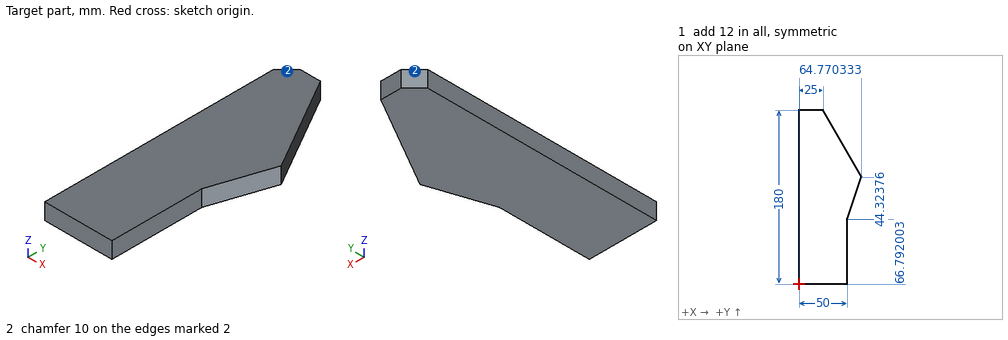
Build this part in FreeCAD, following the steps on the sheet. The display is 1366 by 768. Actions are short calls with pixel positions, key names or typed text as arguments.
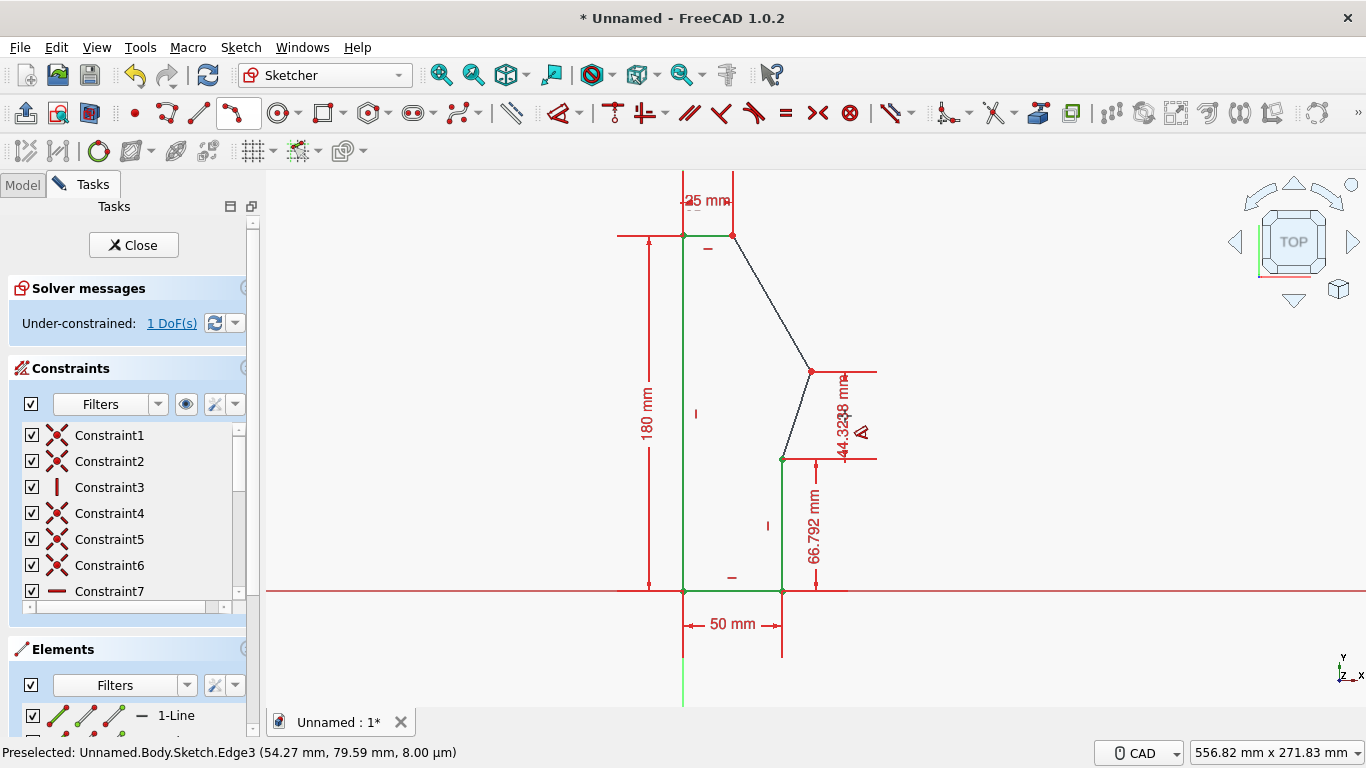
click(811, 372)
click(747, 338)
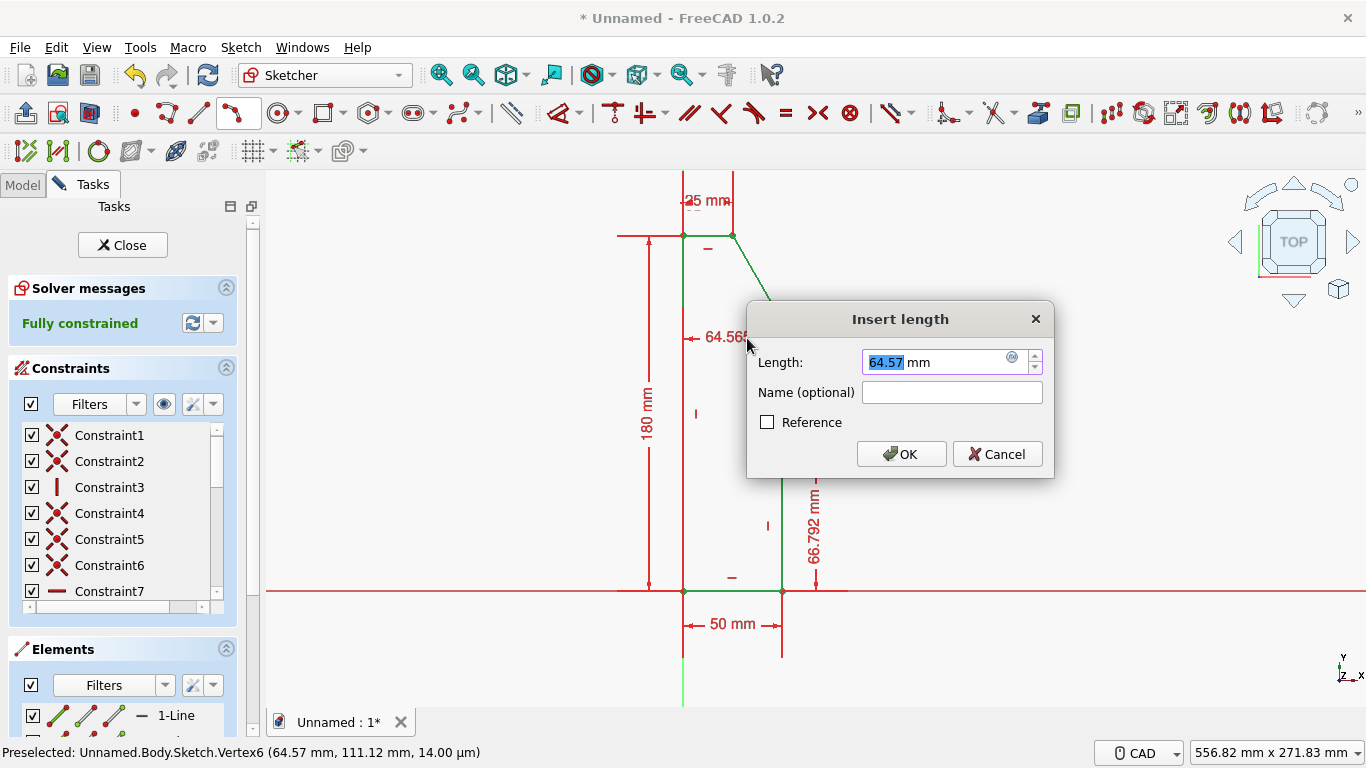
text(64.770333)
key(Return)
key(Escape)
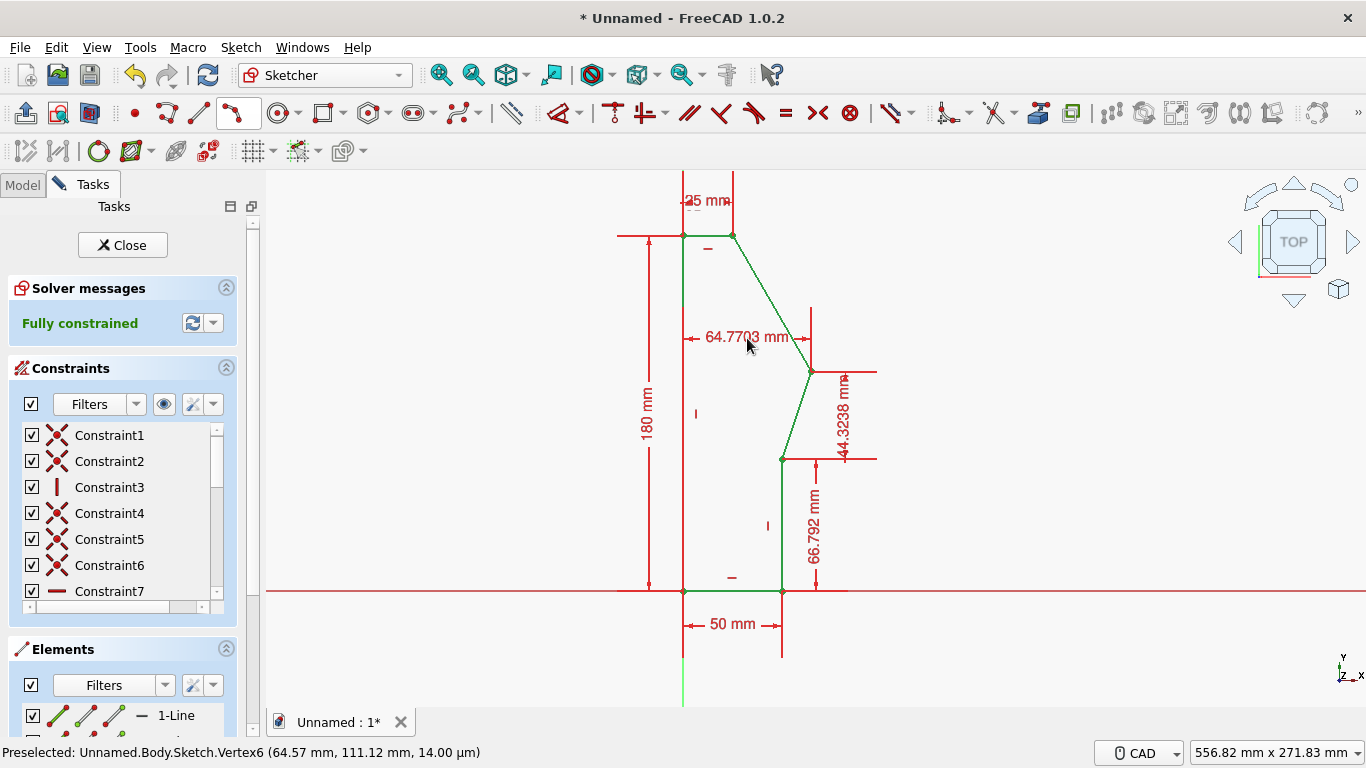
click(123, 245)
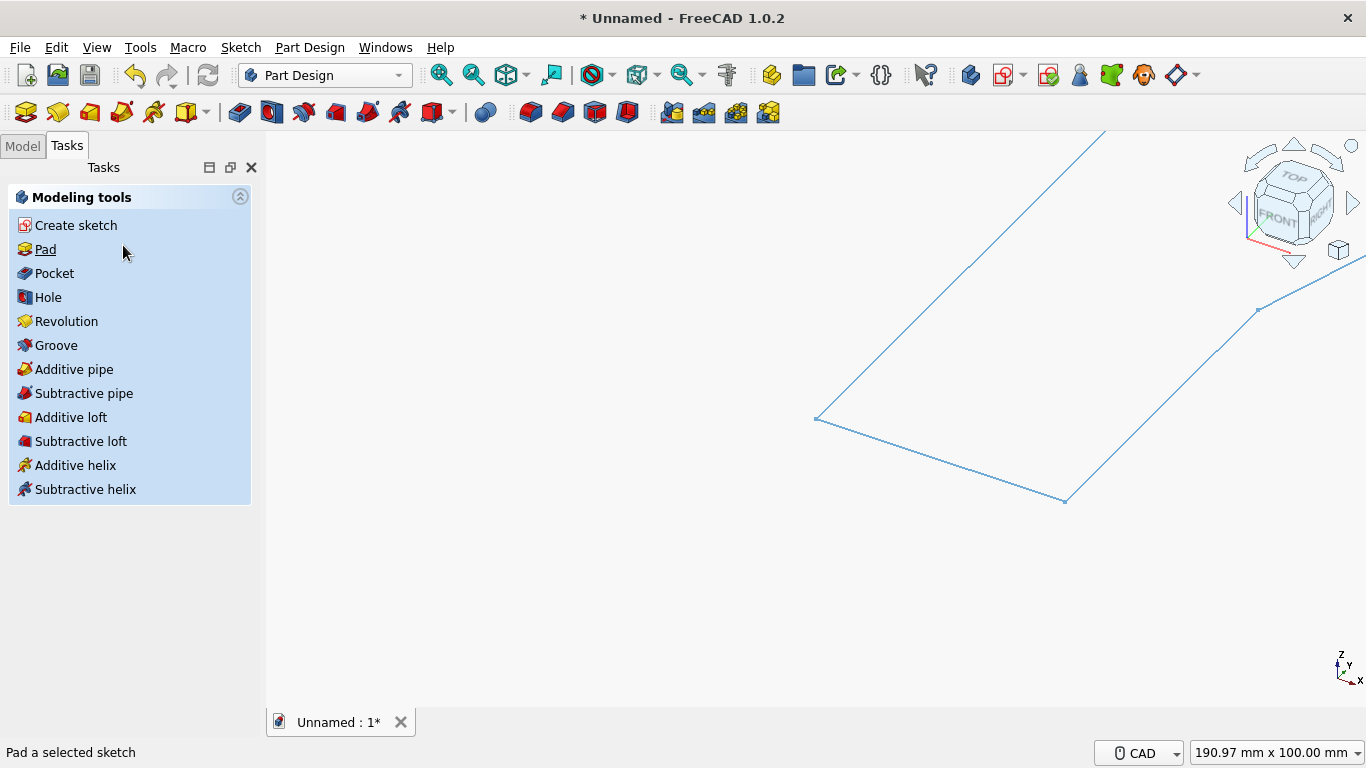
click(26, 112)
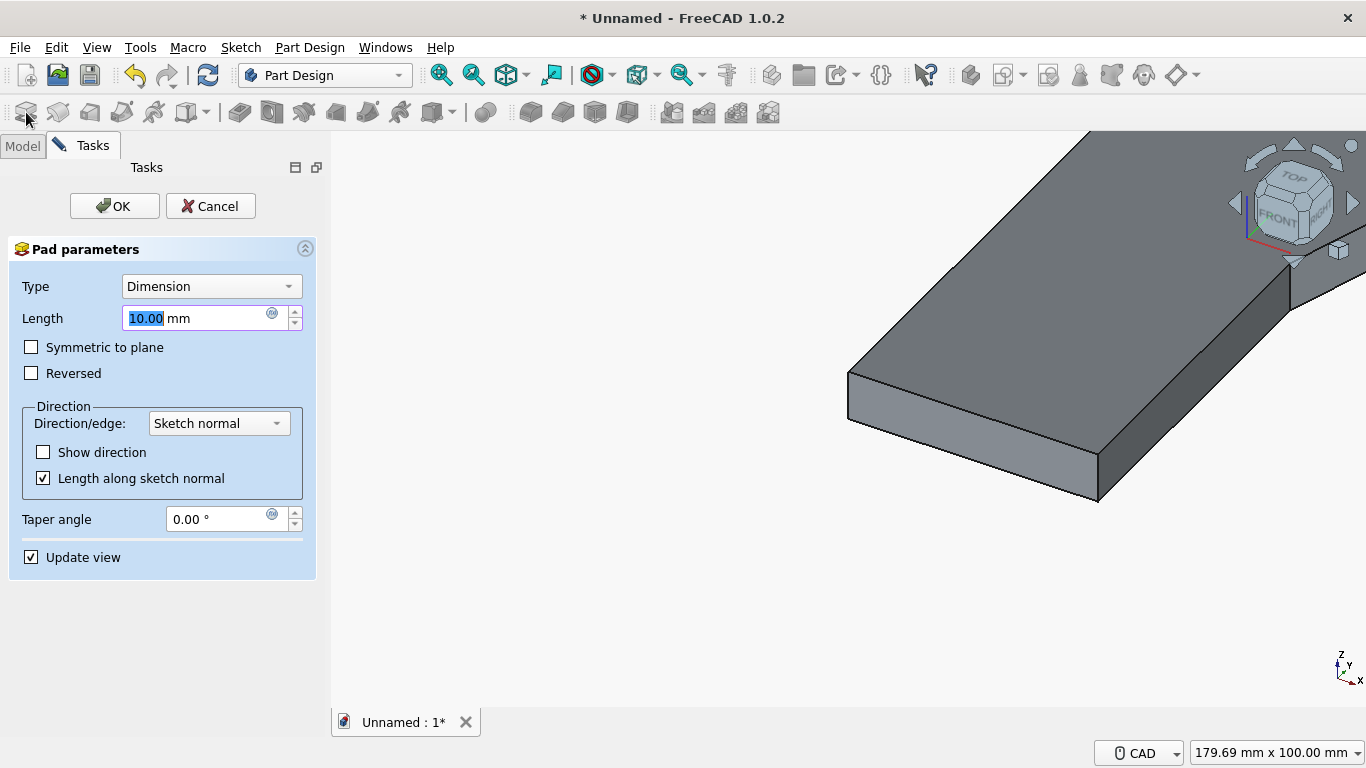
text(12)
key(Tab)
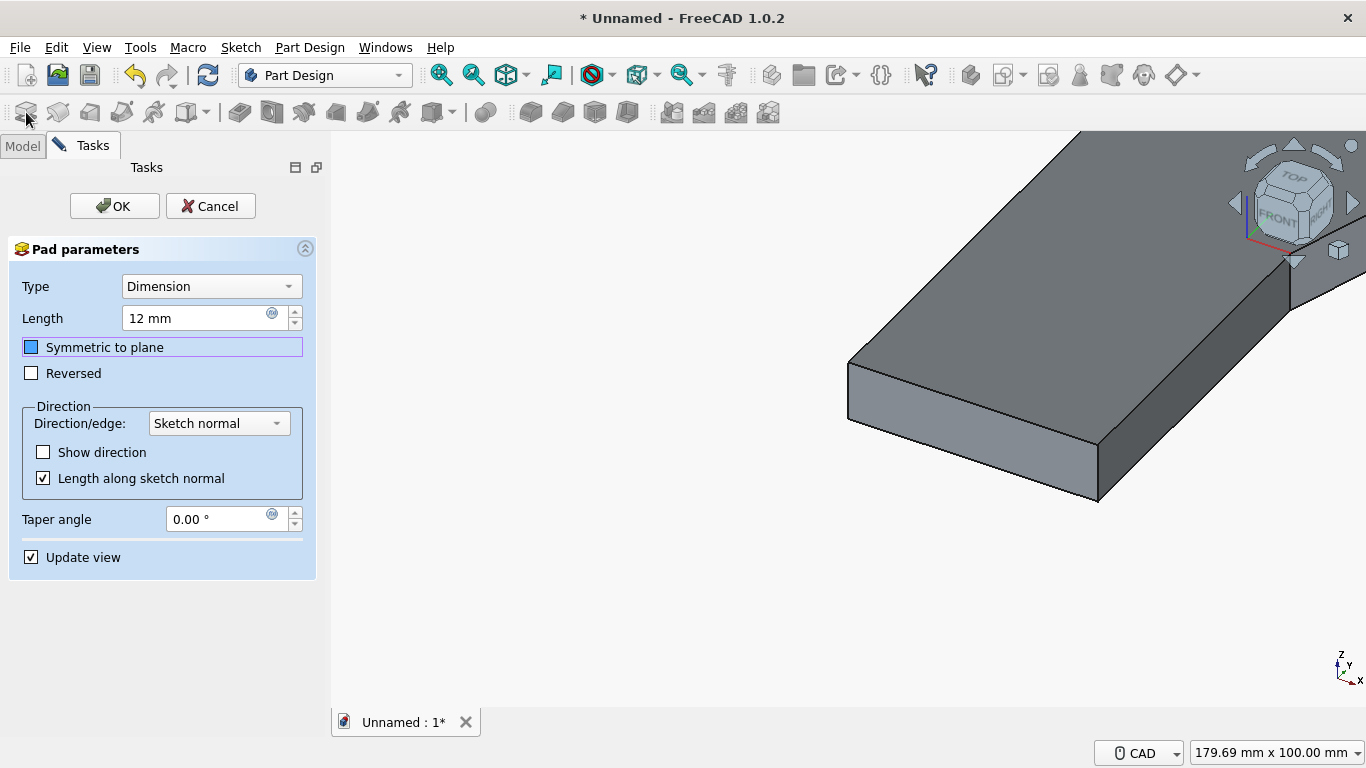
click(30, 347)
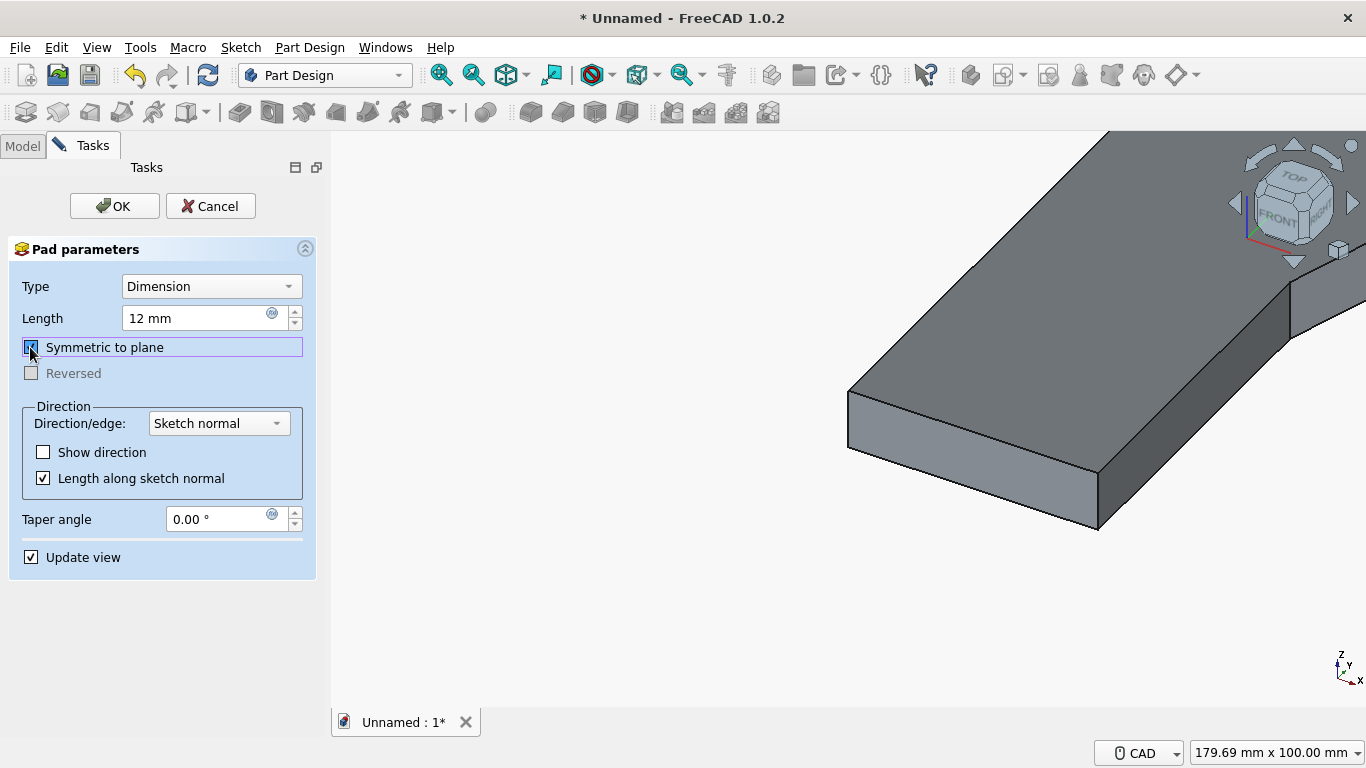
click(115, 206)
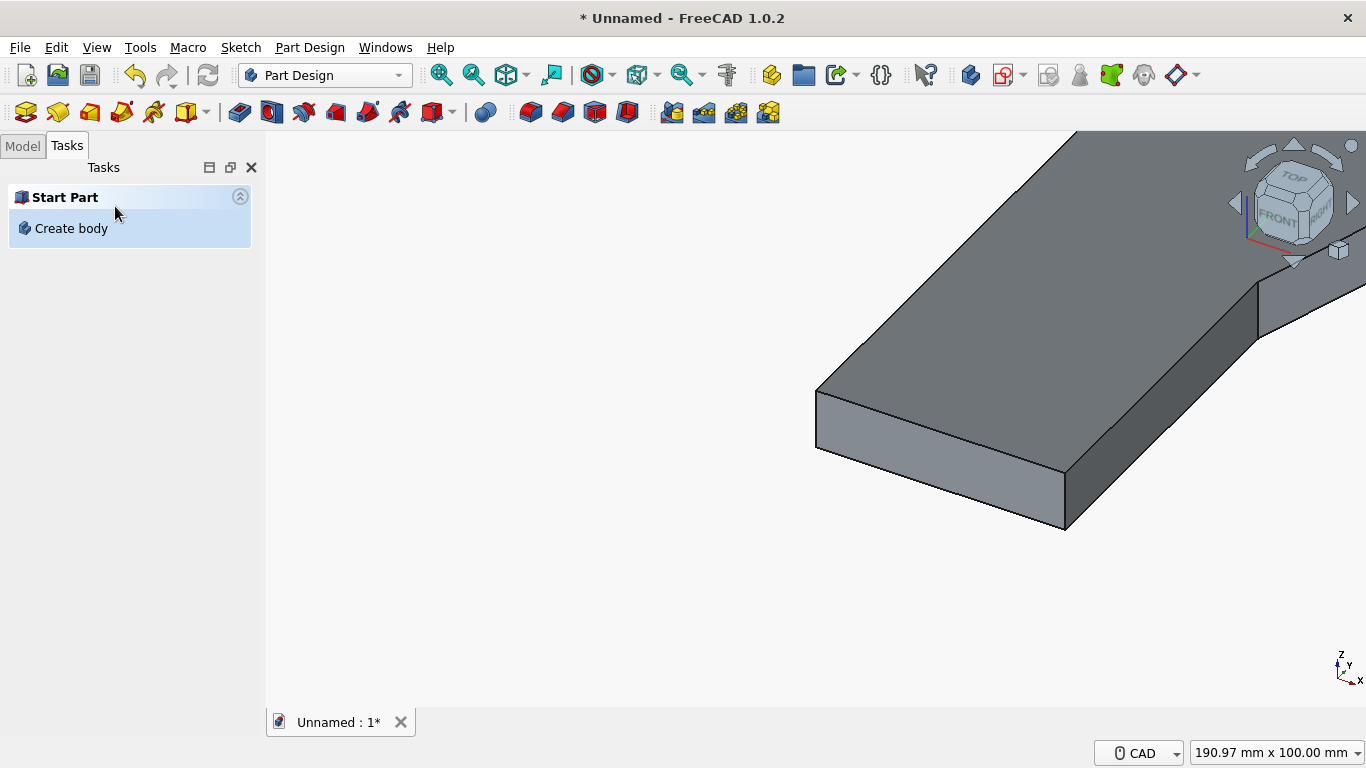
click(442, 76)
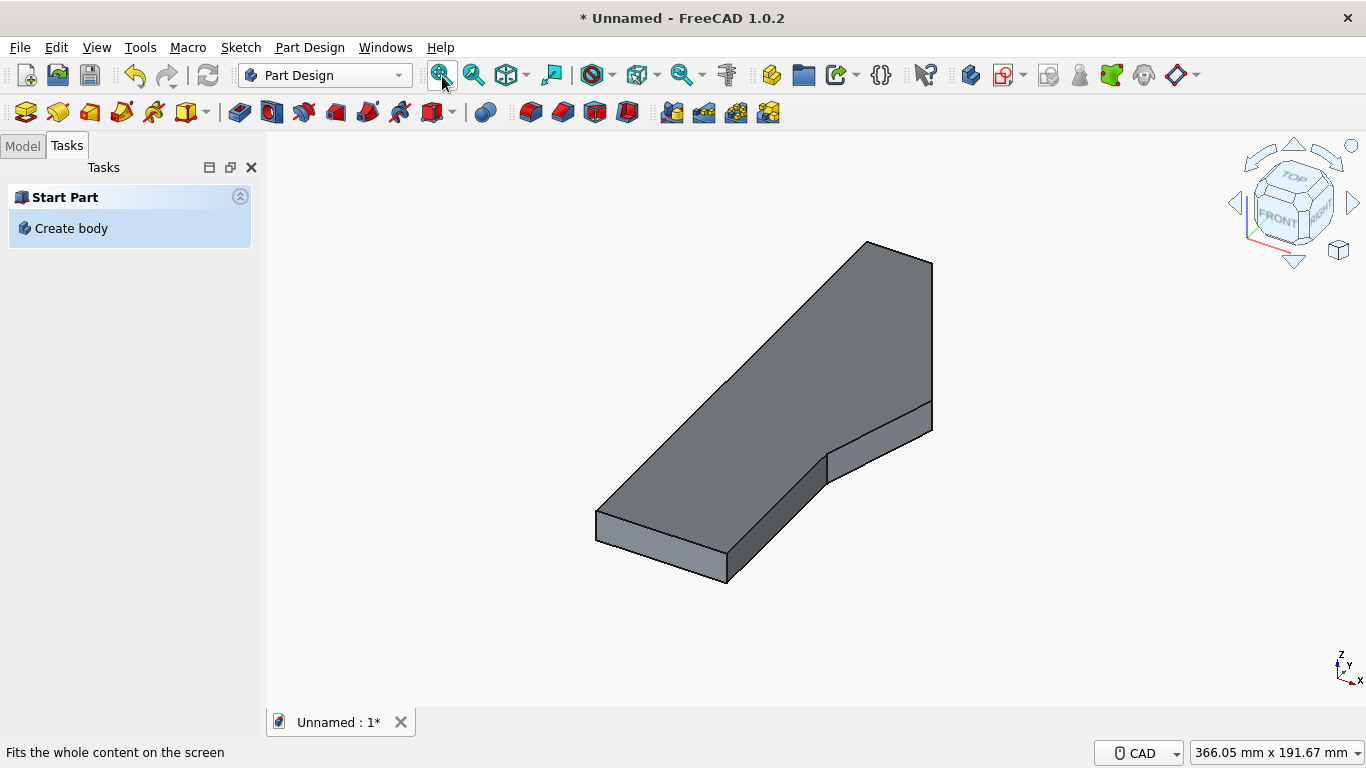
key(0)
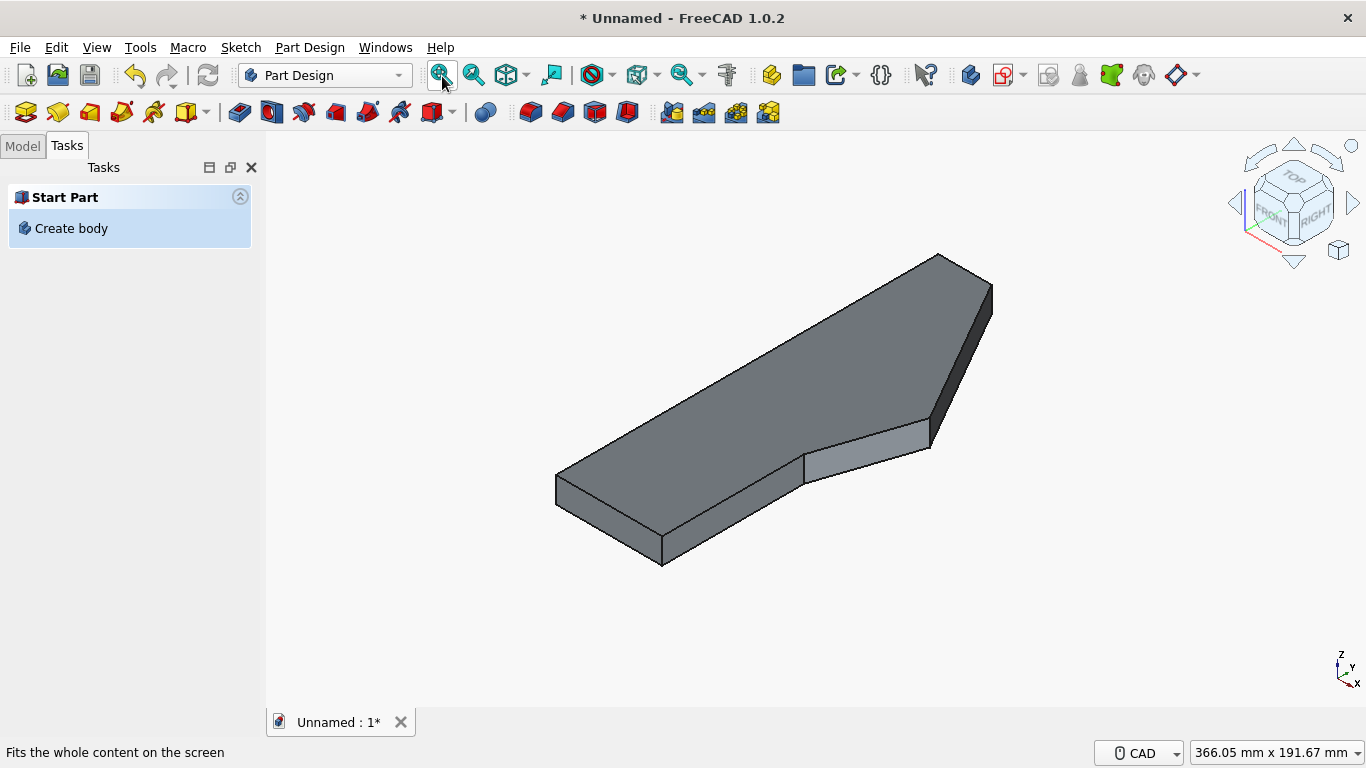
key(2)